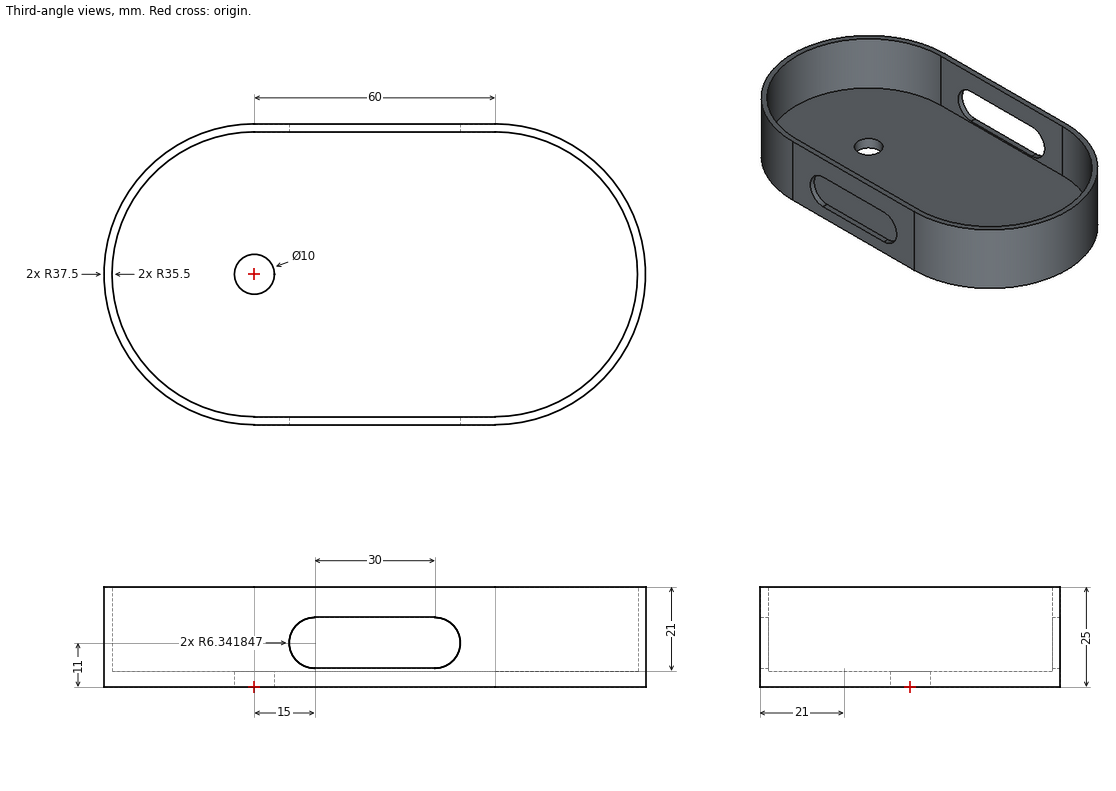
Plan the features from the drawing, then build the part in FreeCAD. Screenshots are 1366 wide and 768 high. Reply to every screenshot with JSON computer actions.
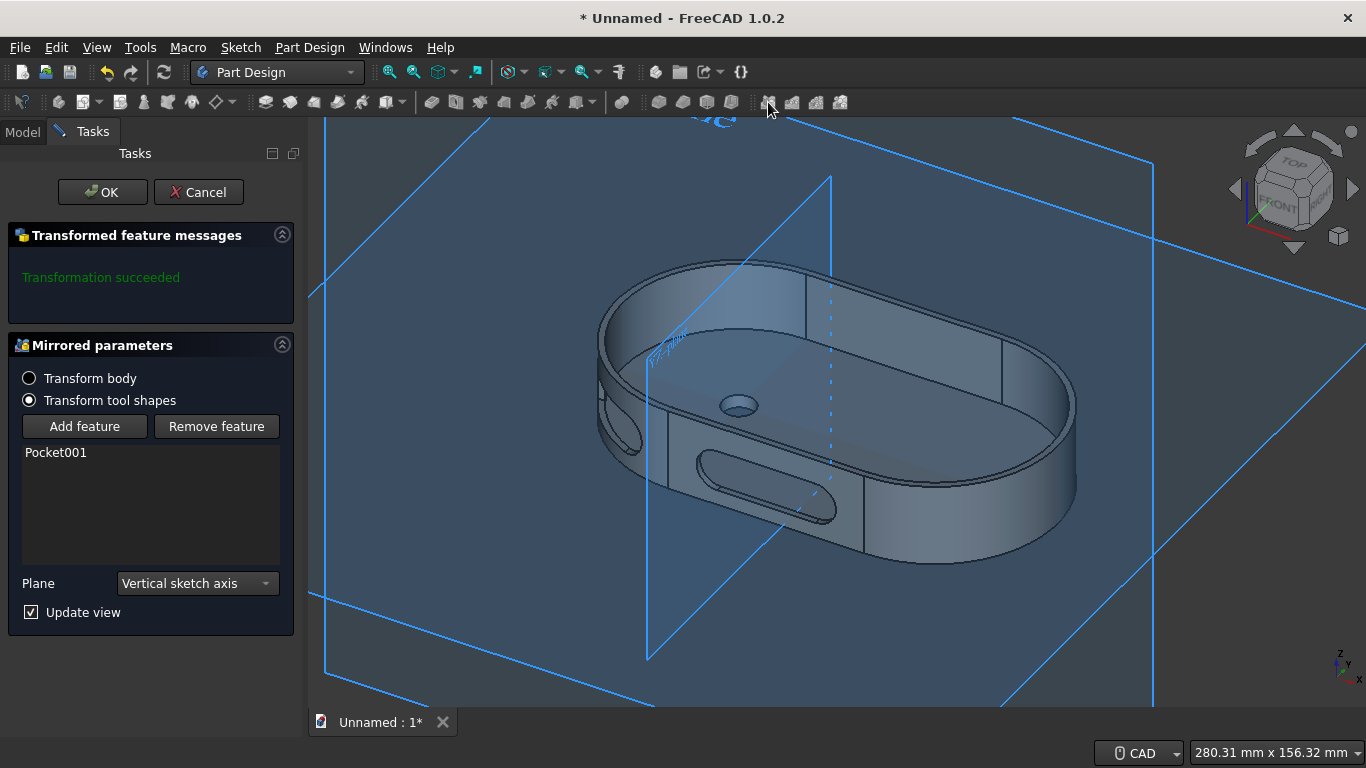
{"action": "left_click", "coordinate": [198, 584]}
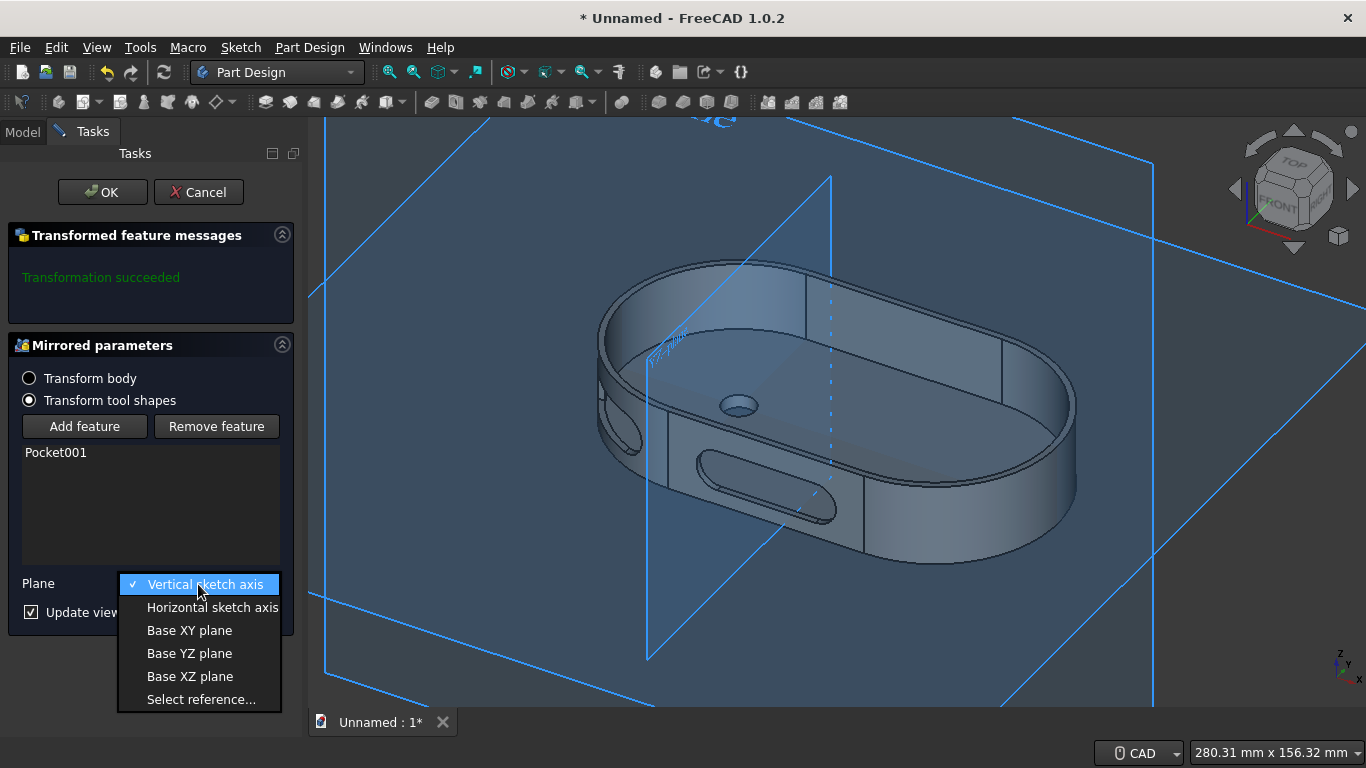
{"action": "left_click", "coordinate": [198, 676]}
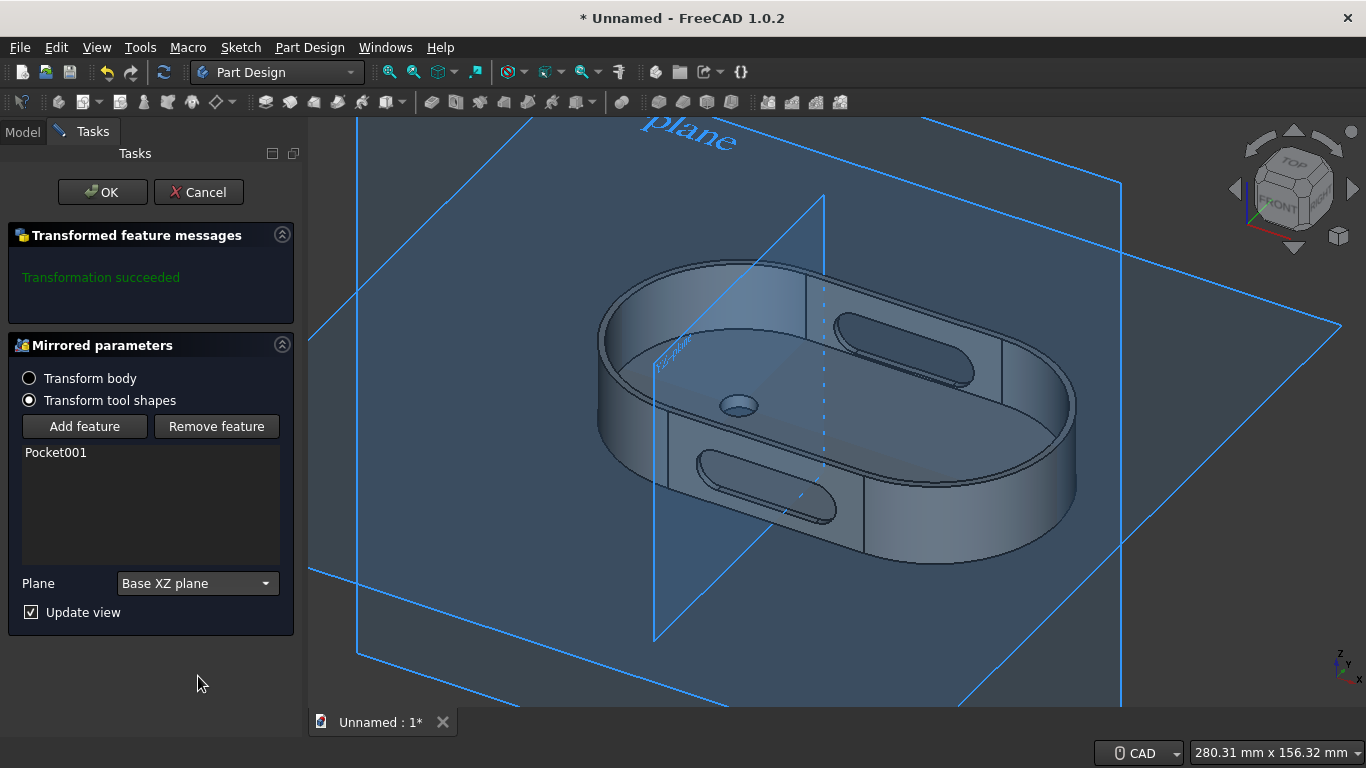
{"action": "left_click", "coordinate": [103, 192]}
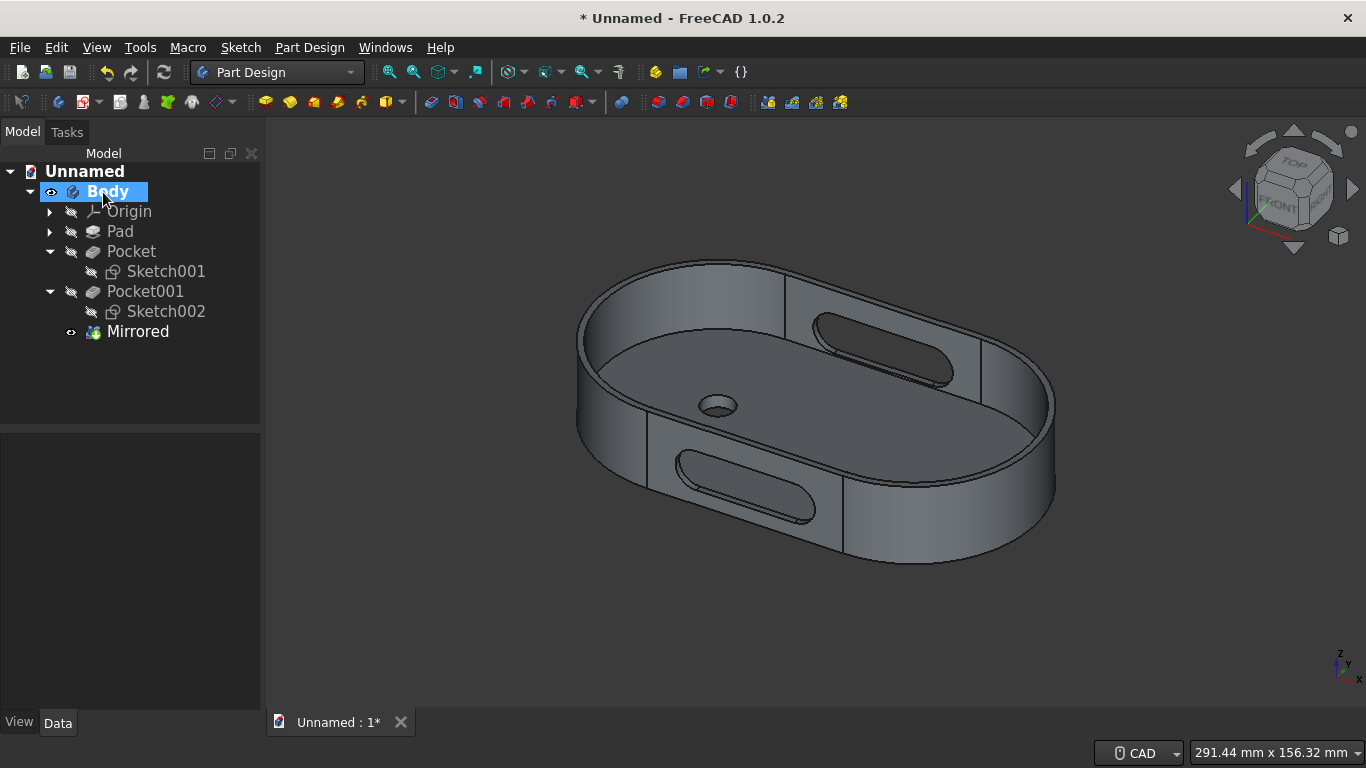
{"action": "key", "text": "0"}